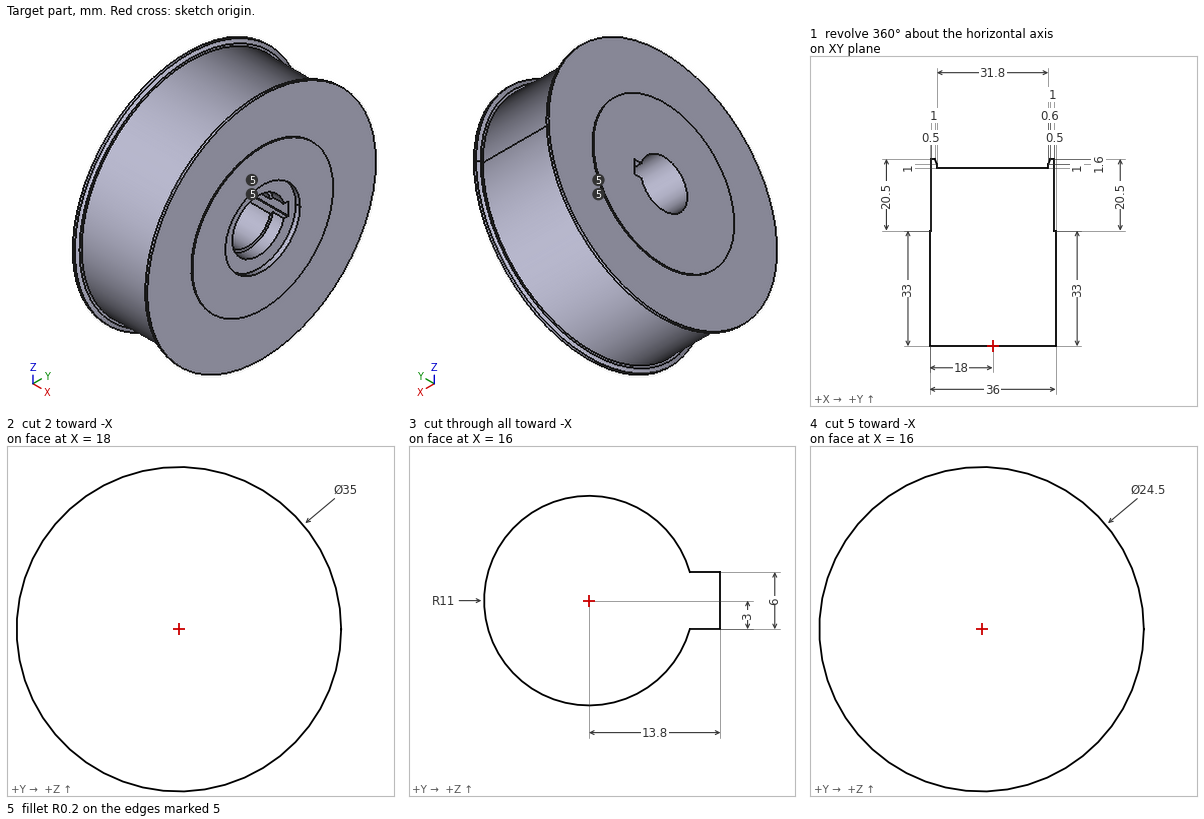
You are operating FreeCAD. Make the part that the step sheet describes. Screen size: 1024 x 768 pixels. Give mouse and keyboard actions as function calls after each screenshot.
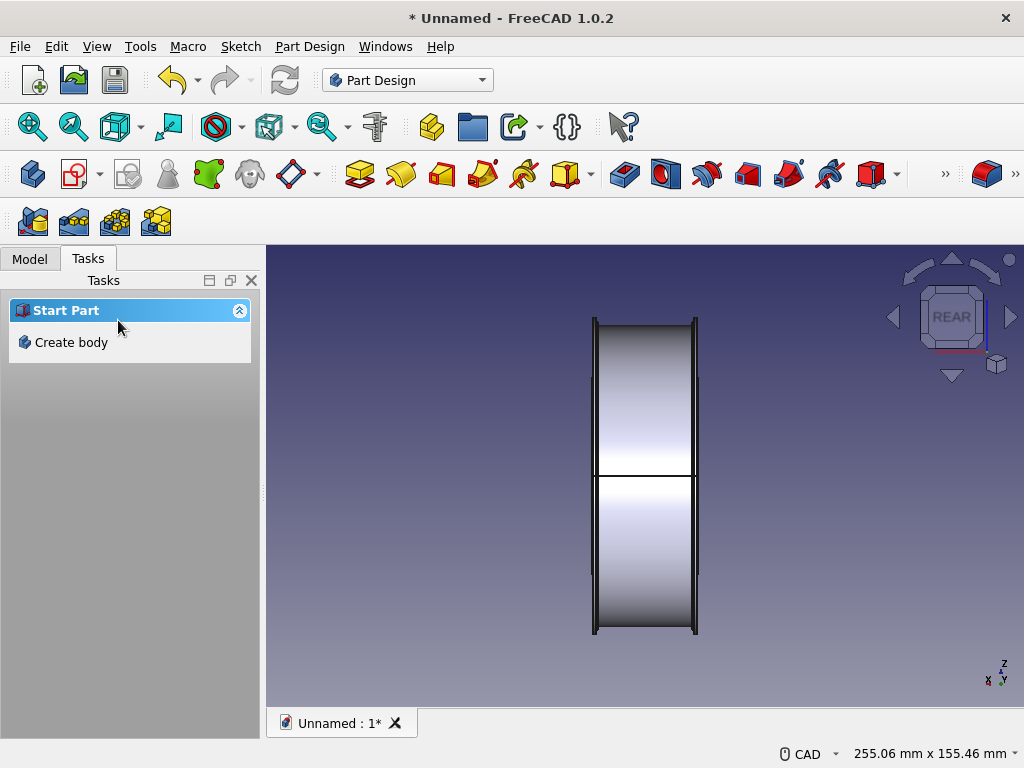
key(6)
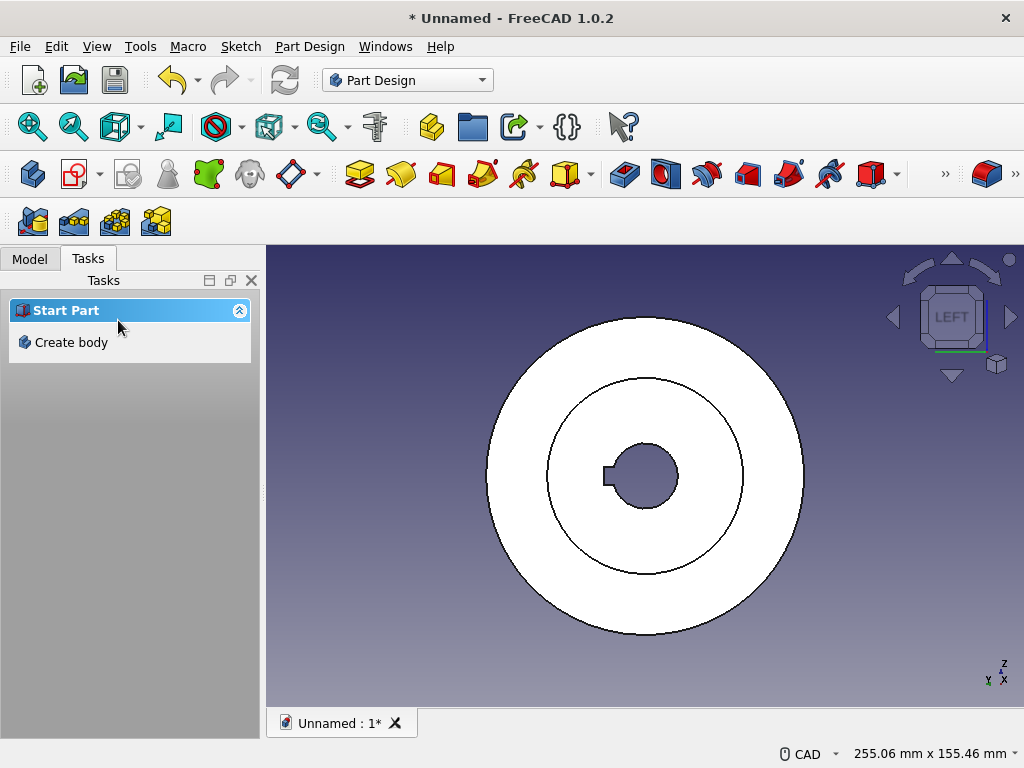
key(v)
key(3)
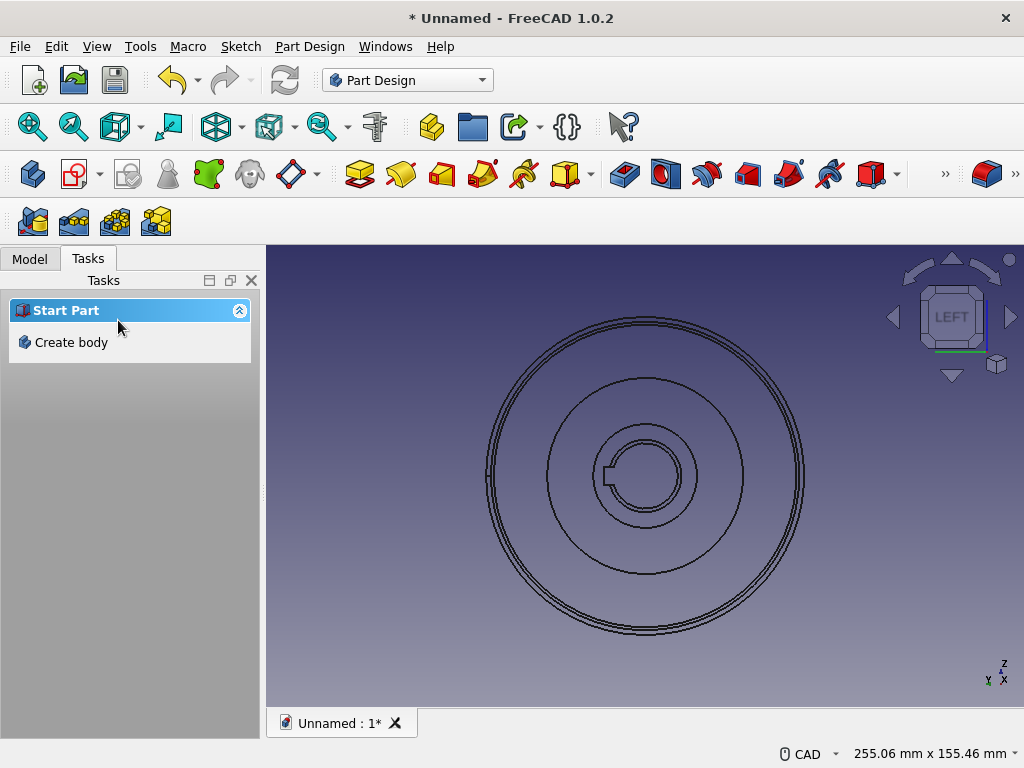
key(0)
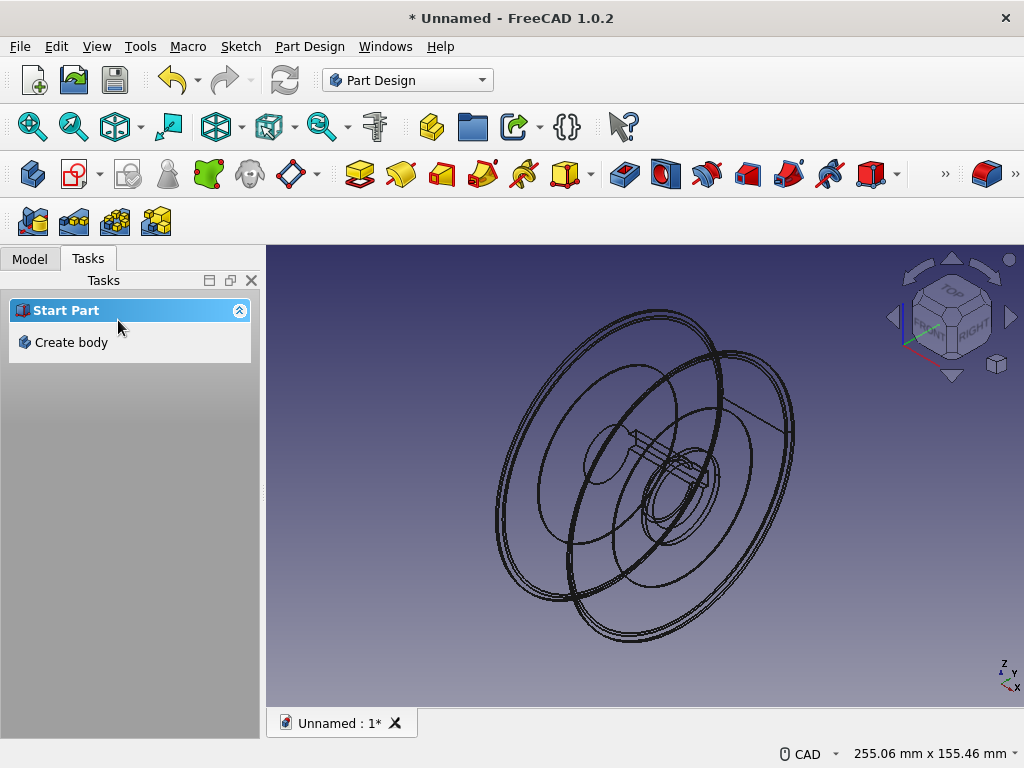
click(665, 446)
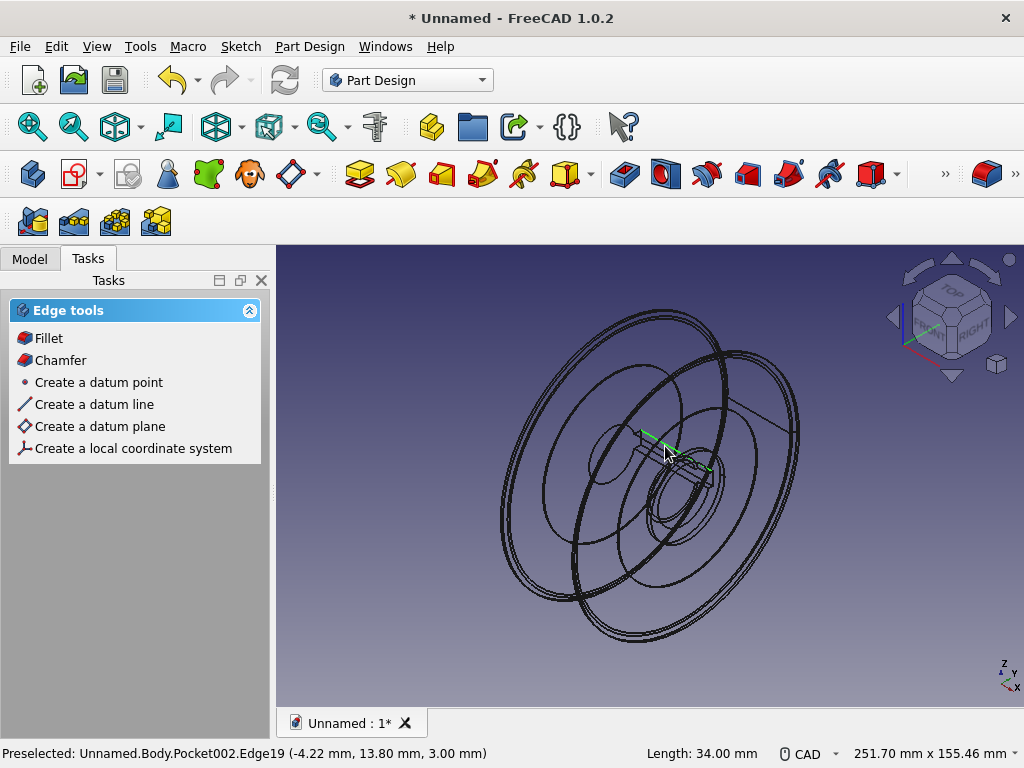
key(2)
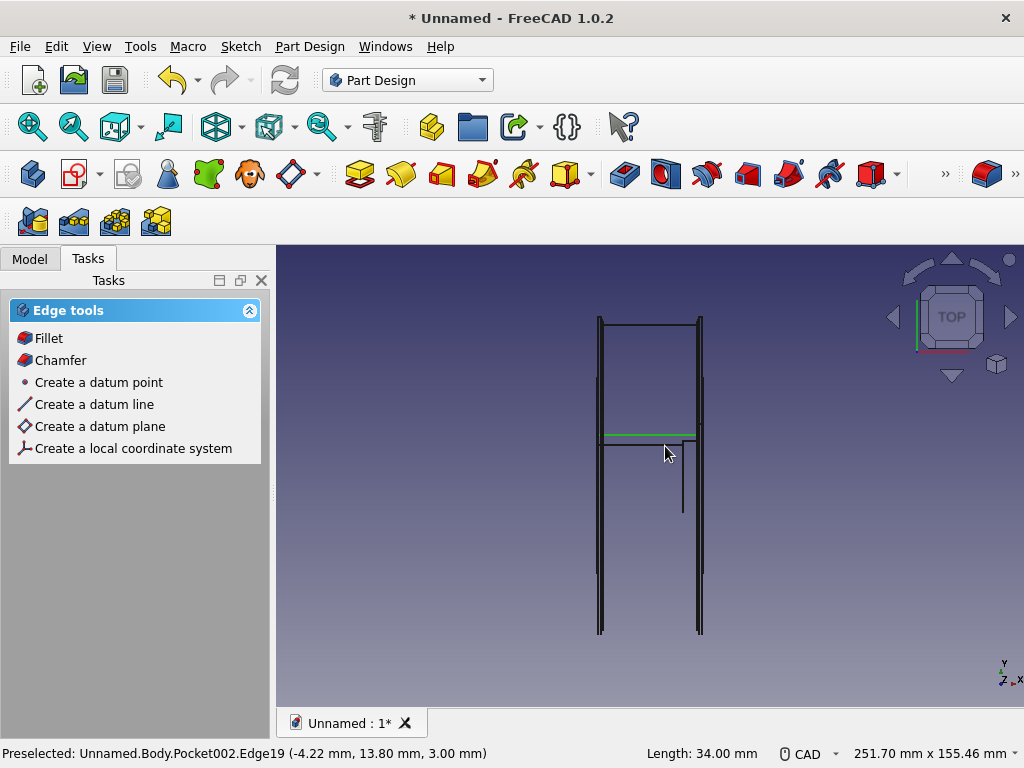
key(1)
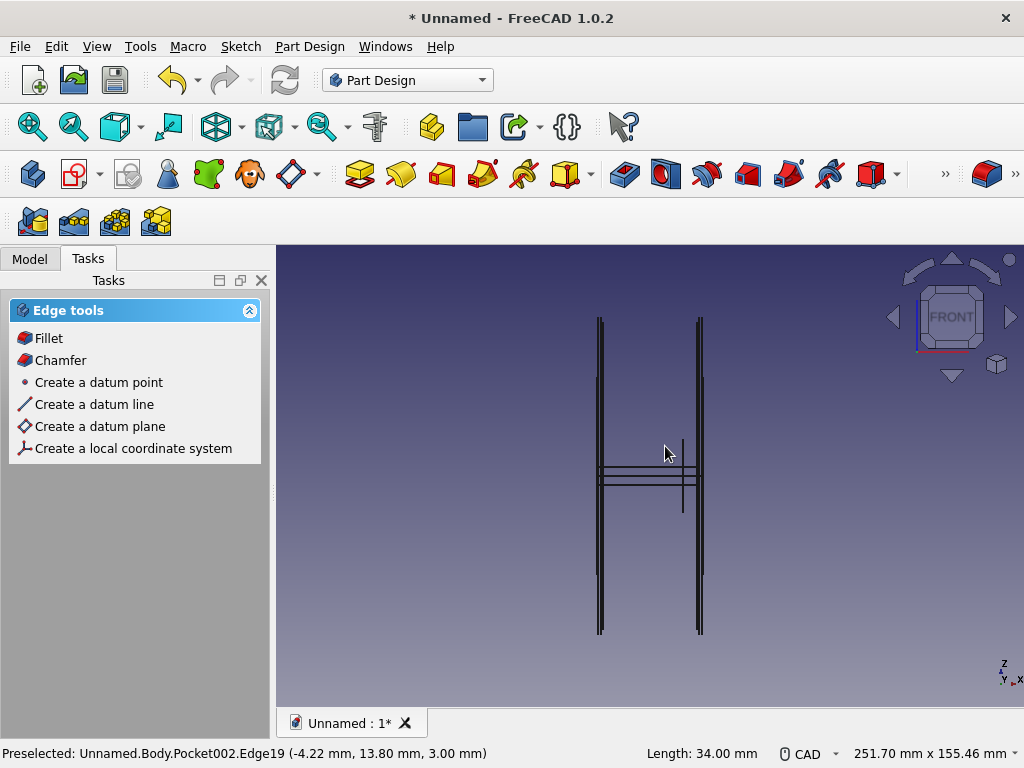
key(3)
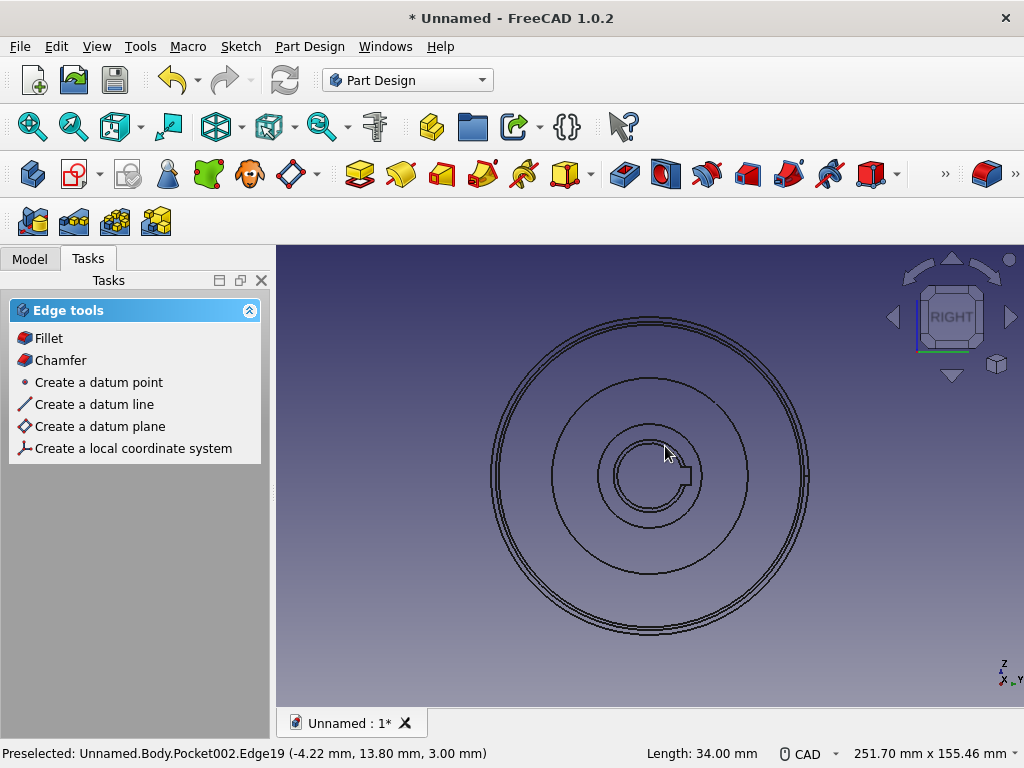
key(5)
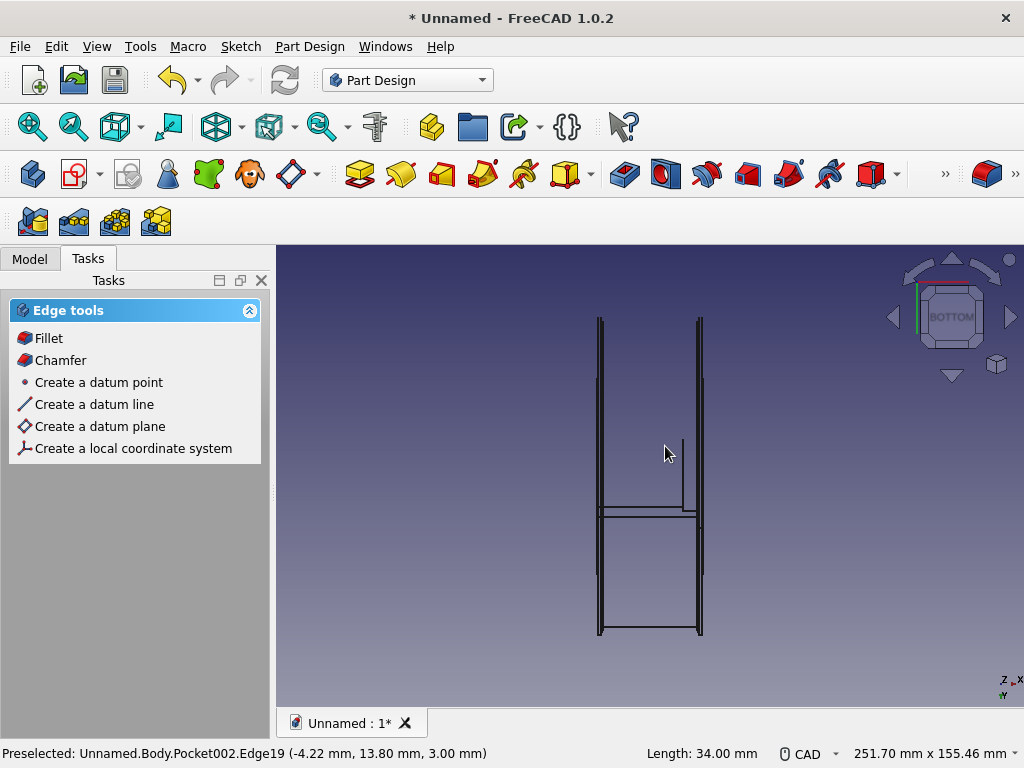
click(647, 516, ctrl)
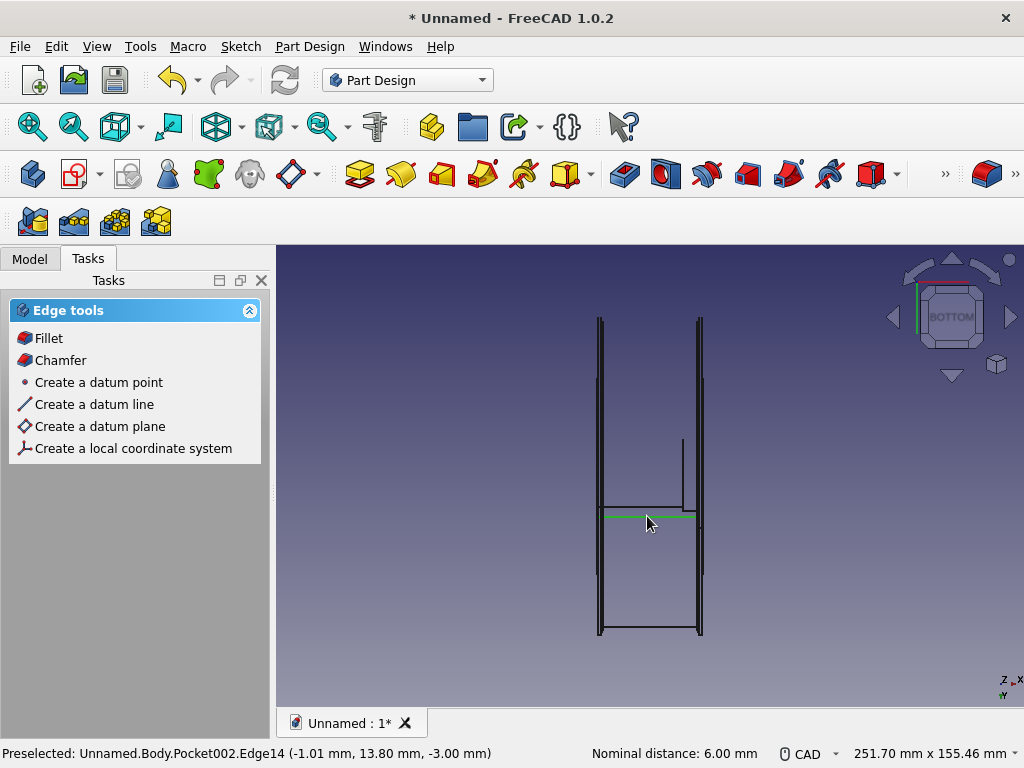
key(v)
key(1)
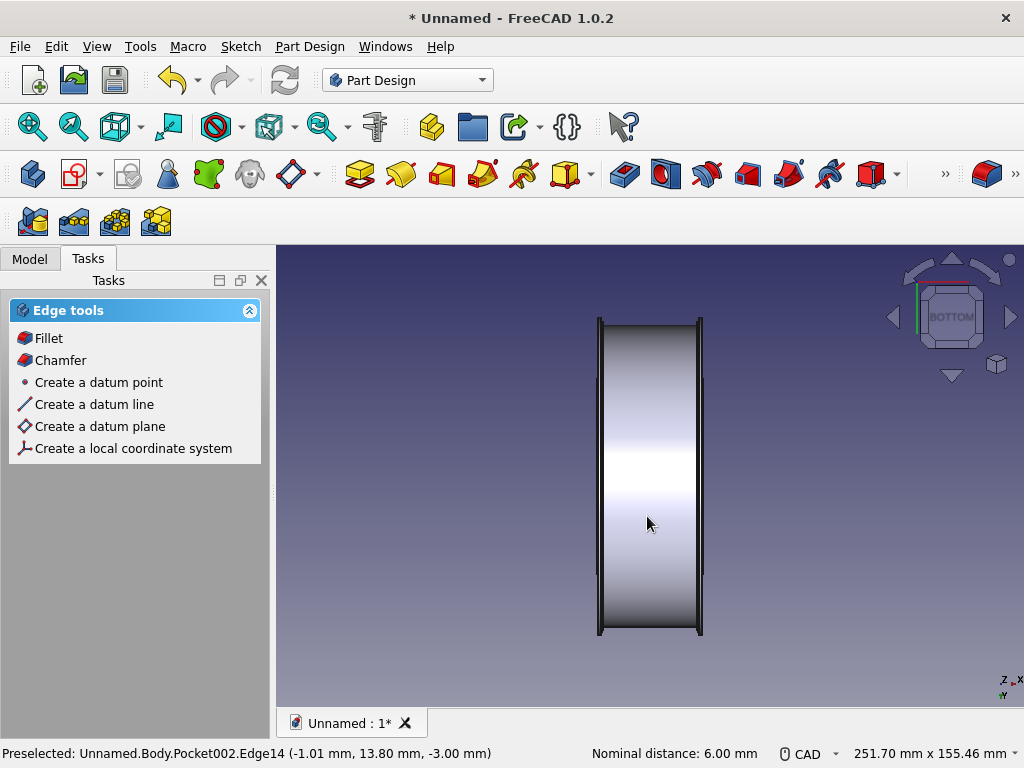
click(987, 174)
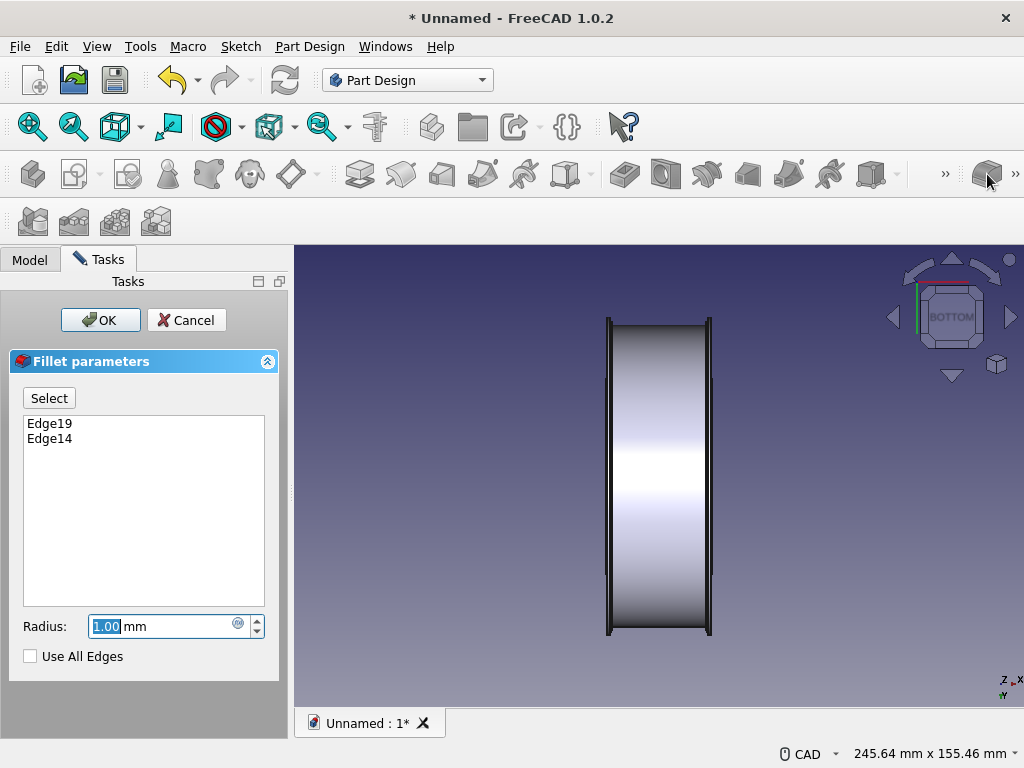
text(0.2)
key(Tab)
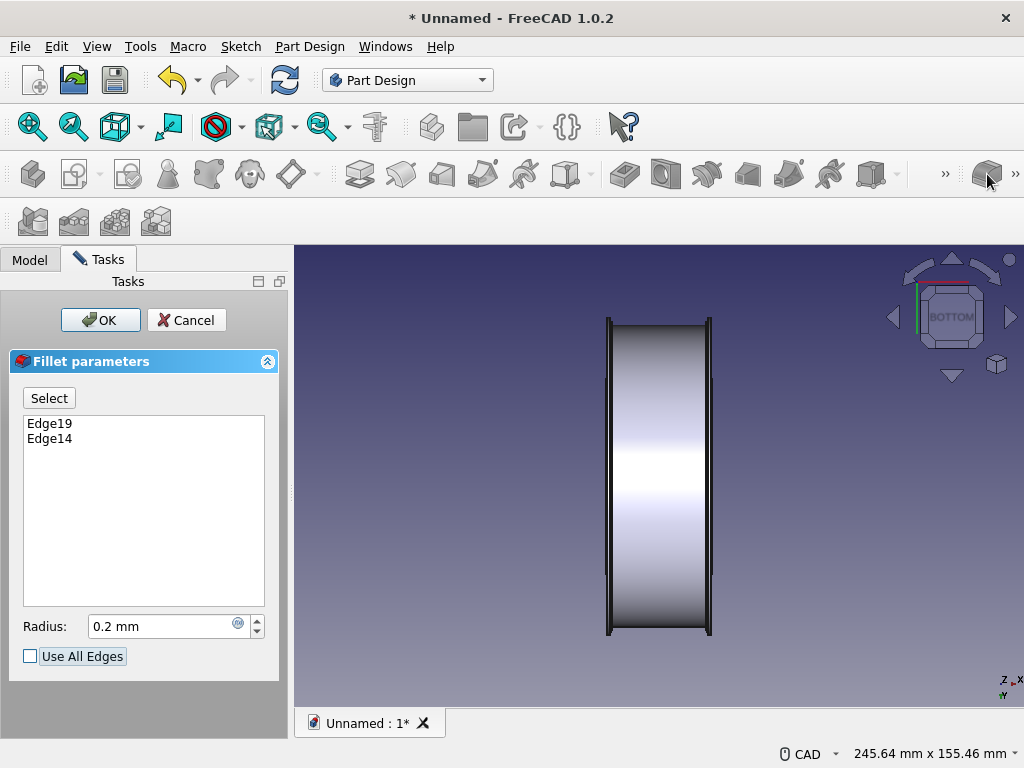
click(101, 320)